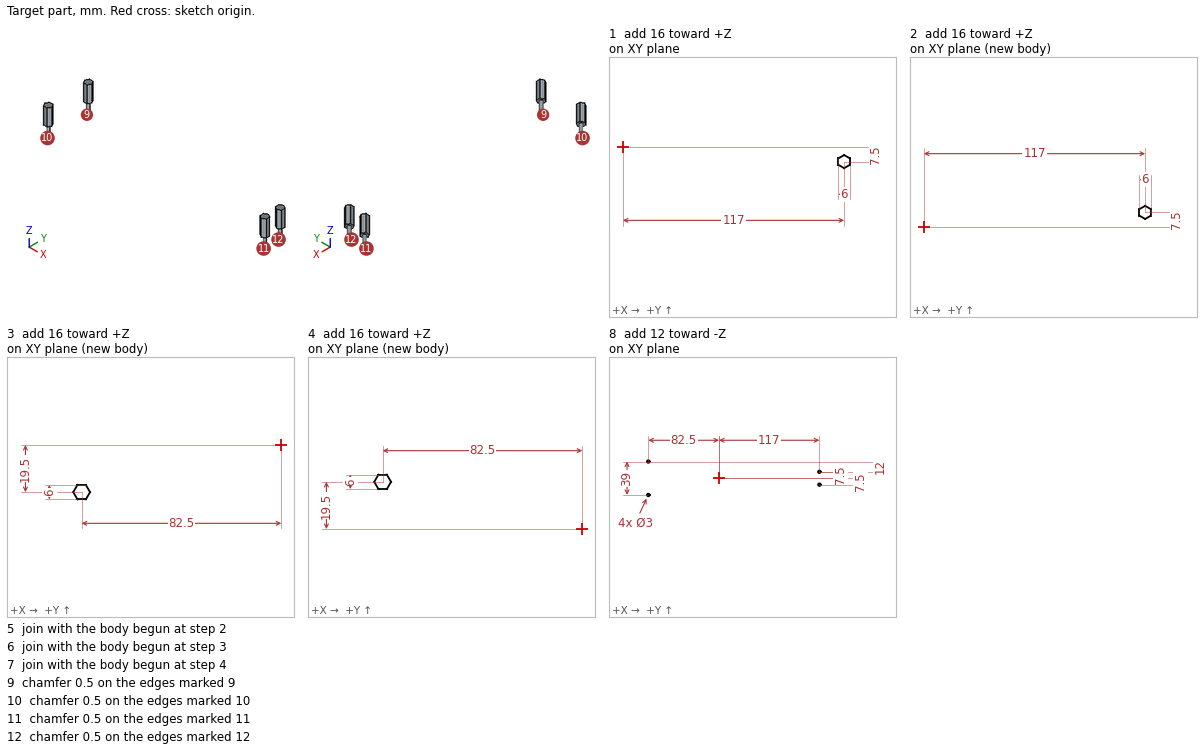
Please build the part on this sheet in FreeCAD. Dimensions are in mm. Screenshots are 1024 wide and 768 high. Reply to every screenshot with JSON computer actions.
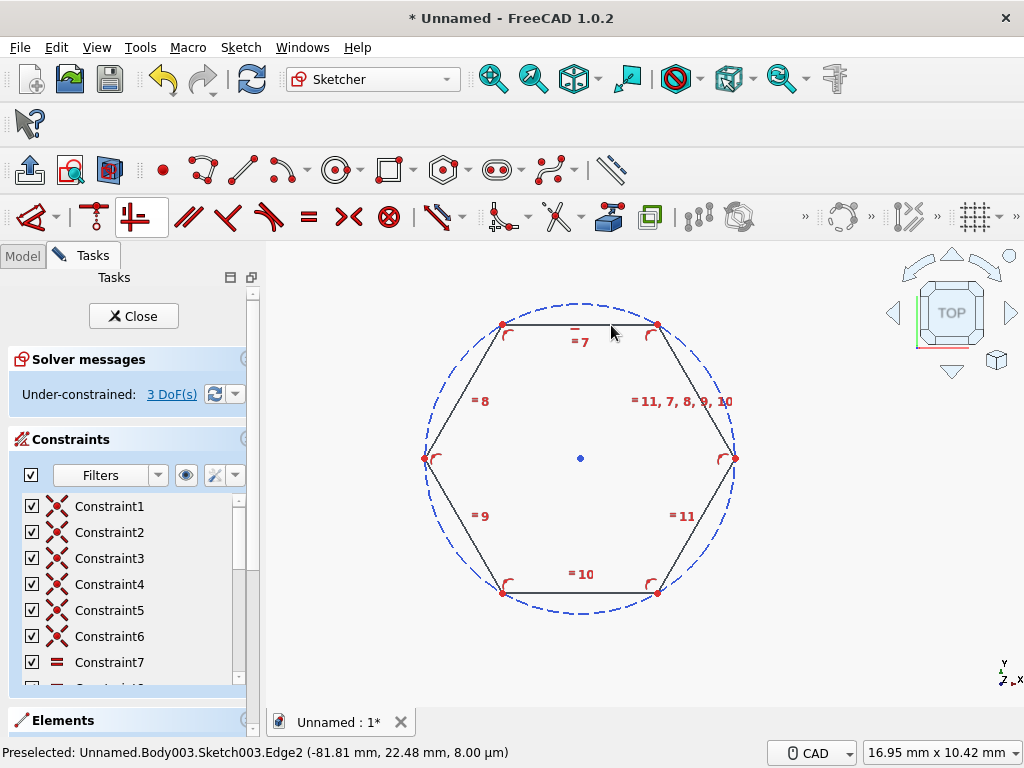
{"action": "left_click", "coordinate": [32, 218]}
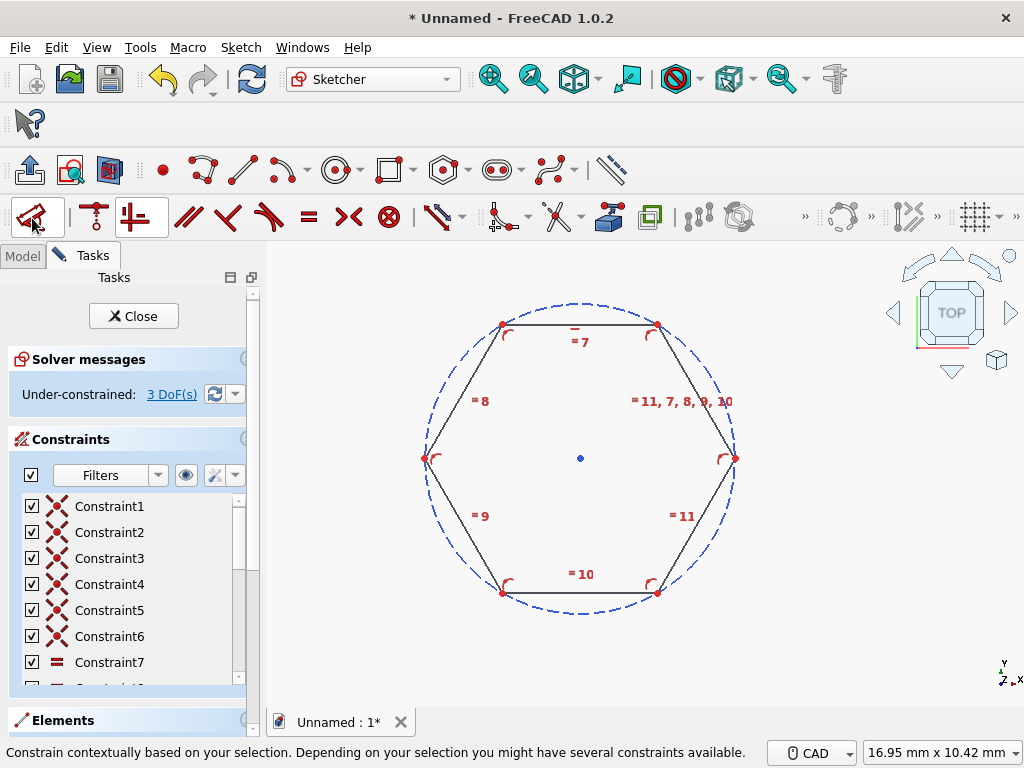
{"action": "left_click", "coordinate": [502, 593]}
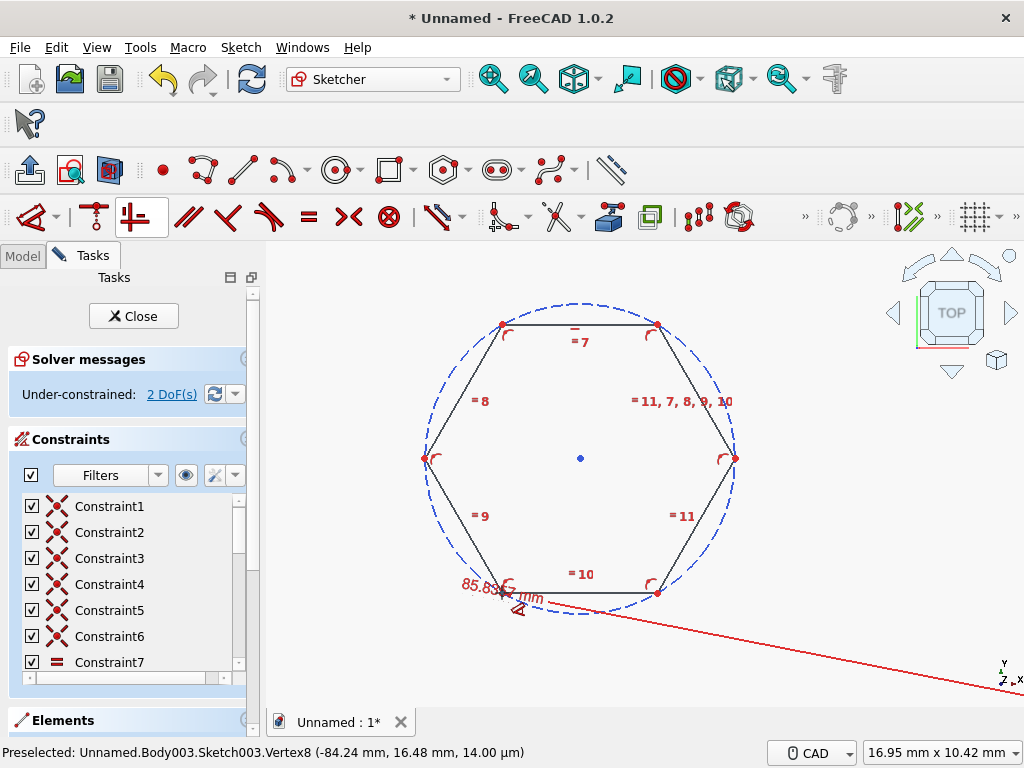
{"action": "left_click", "coordinate": [657, 325]}
{"action": "left_click", "coordinate": [468, 459]}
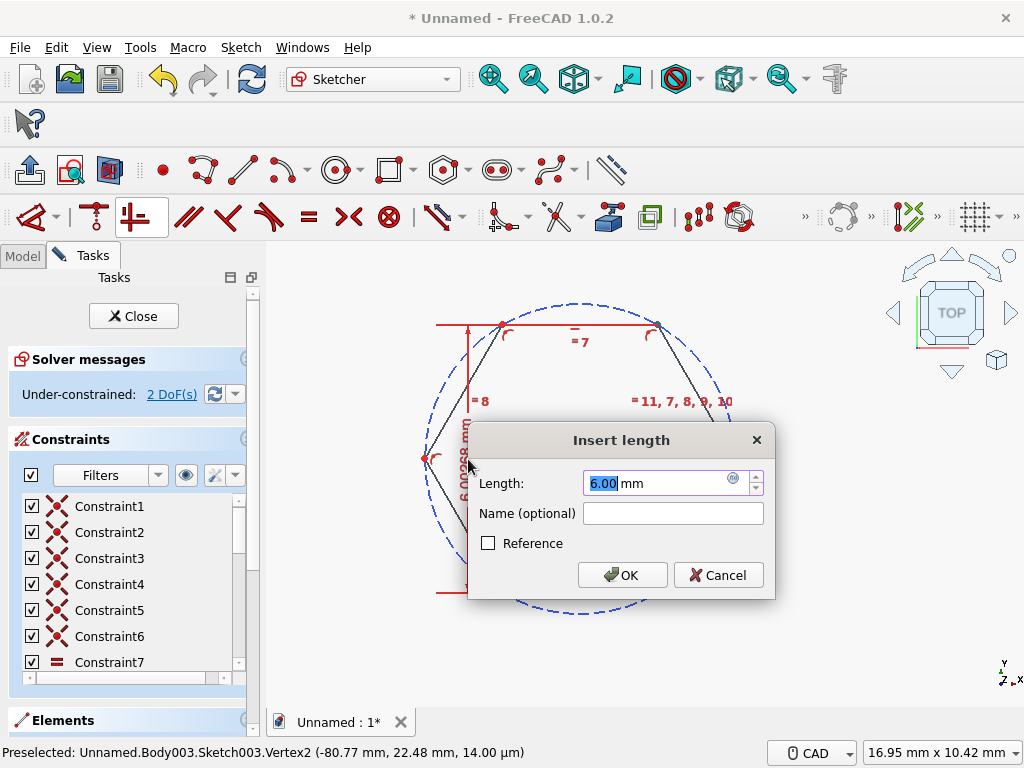
{"action": "type", "text": "6"}
{"action": "key", "text": "Return"}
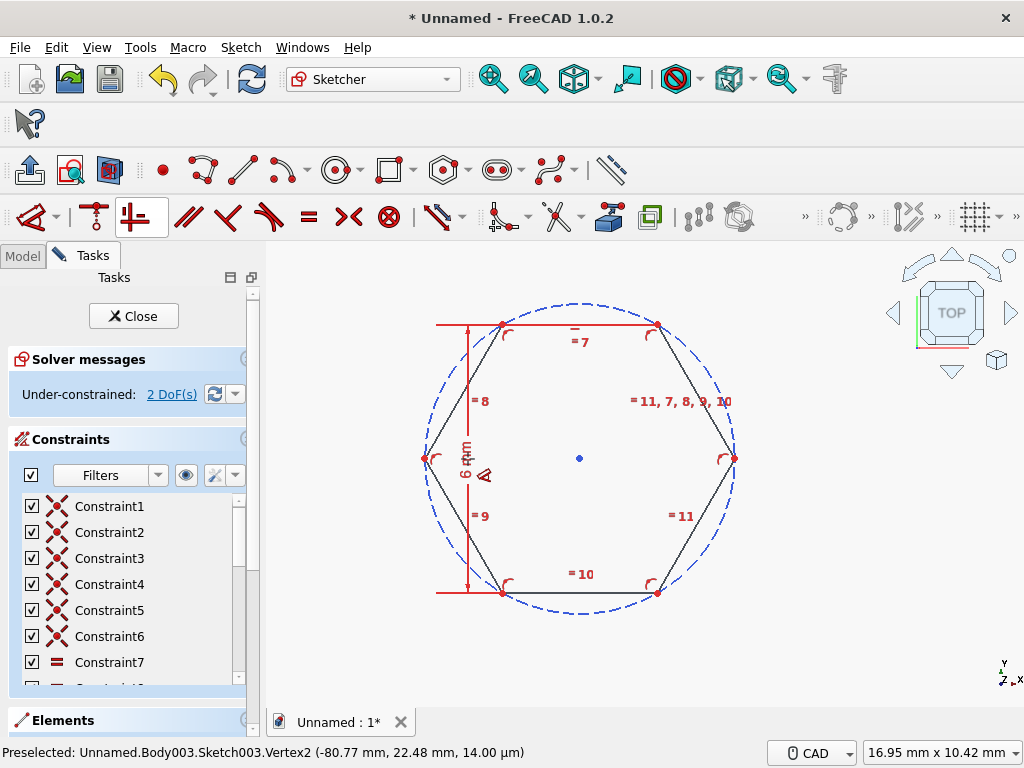
{"action": "left_click", "coordinate": [580, 459]}
{"action": "left_click", "coordinate": [655, 425]}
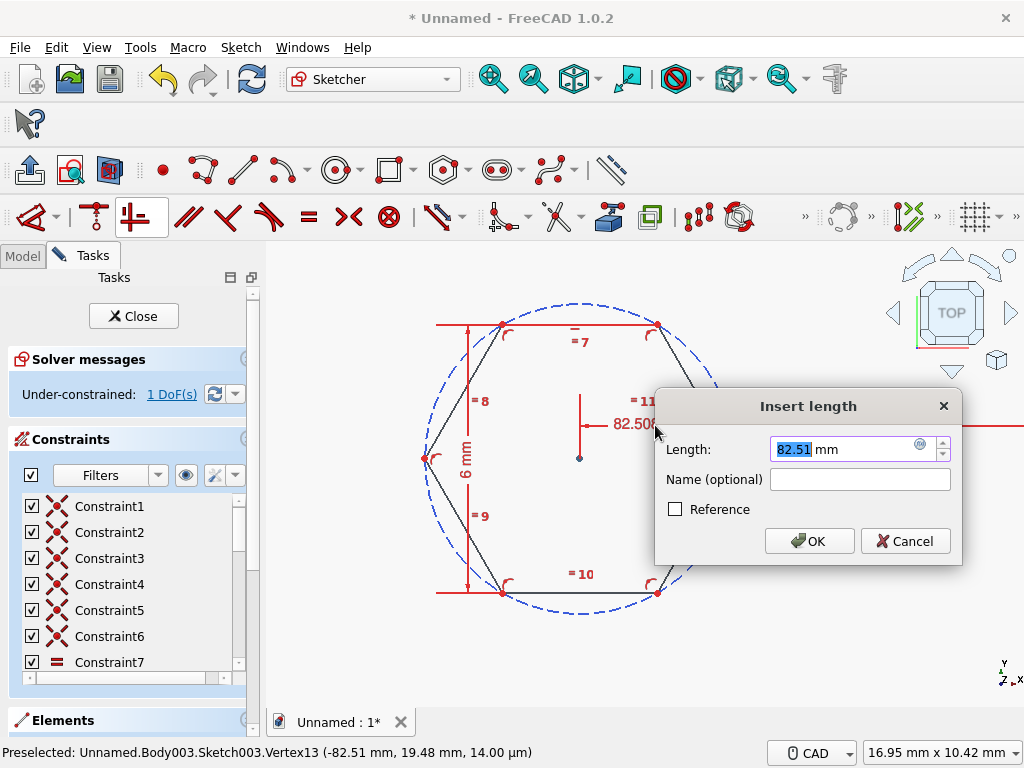
{"action": "type", "text": "82.5"}
{"action": "key", "text": "Return"}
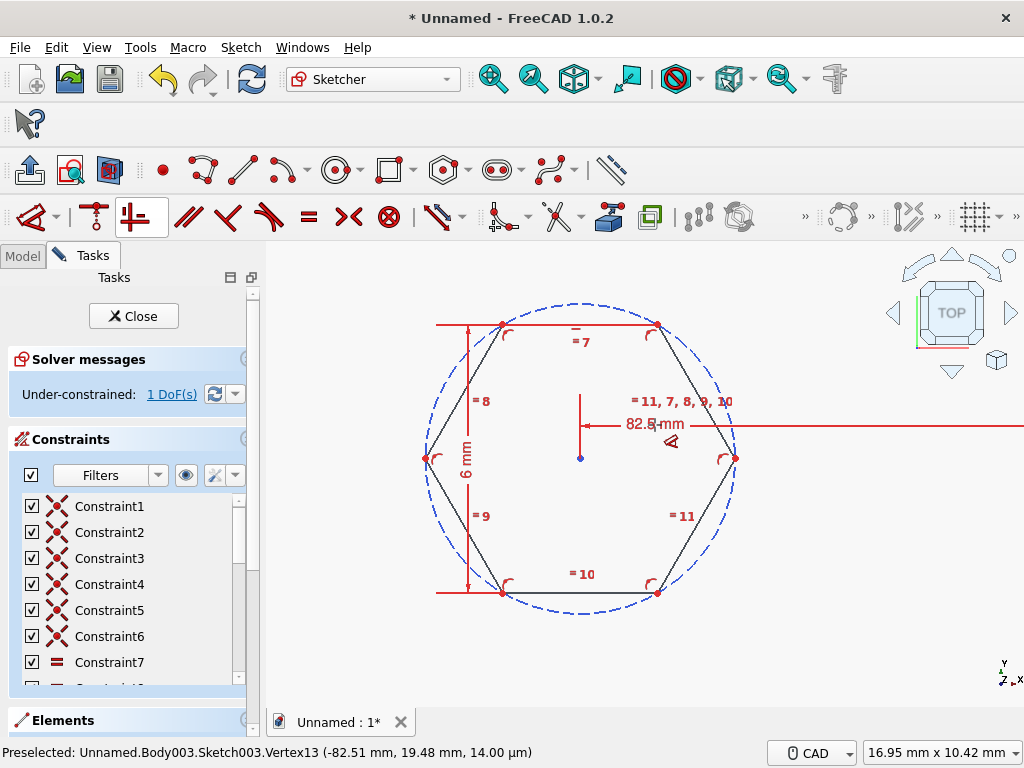
{"action": "left_click", "coordinate": [580, 459]}
{"action": "left_click", "coordinate": [546, 569]}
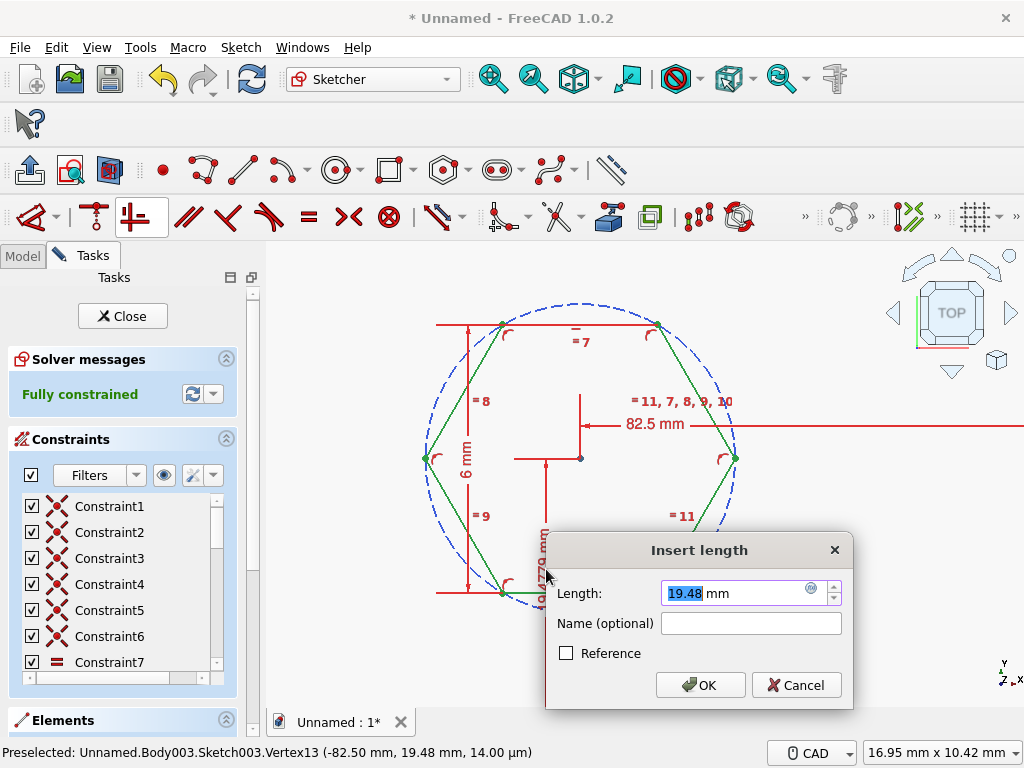
{"action": "type", "text": "19.5"}
{"action": "key", "text": "Return"}
{"action": "key", "text": "Escape"}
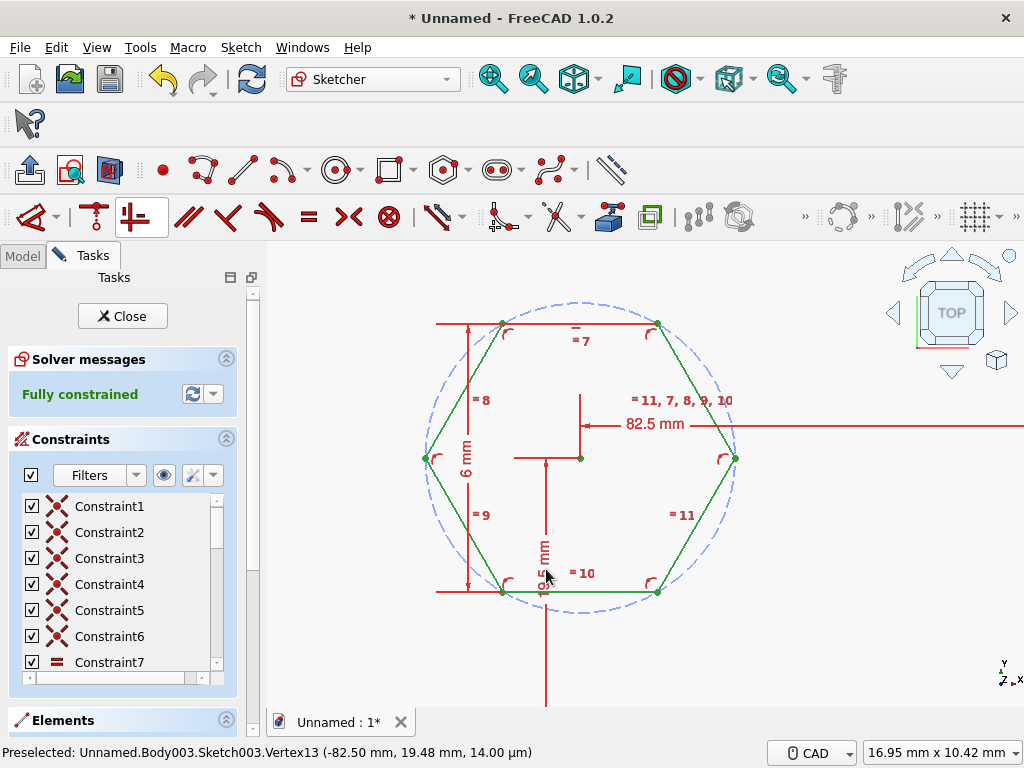
{"action": "left_click", "coordinate": [123, 316]}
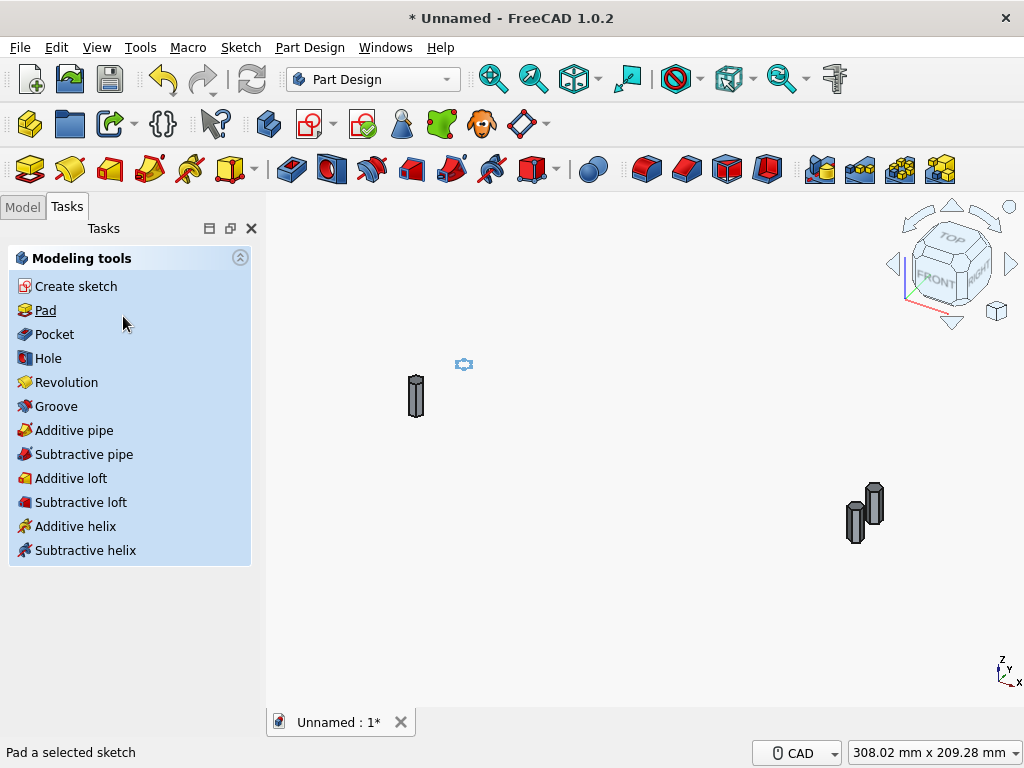
{"action": "left_click", "coordinate": [30, 170]}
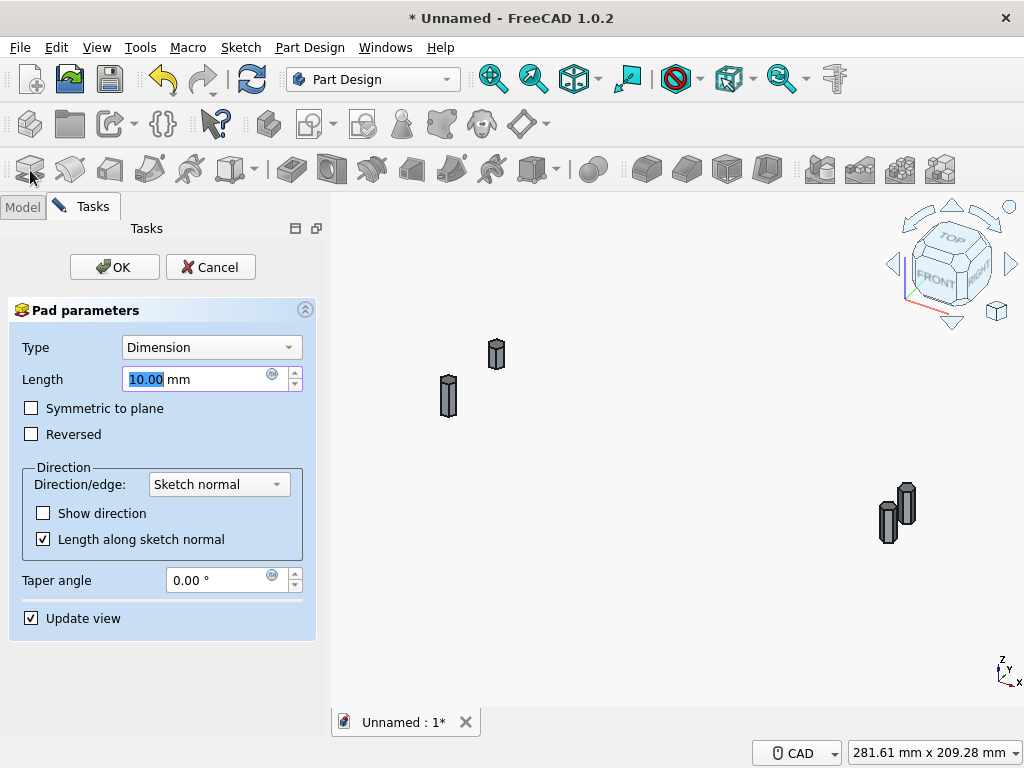
{"action": "type", "text": "16"}
{"action": "key", "text": "Tab"}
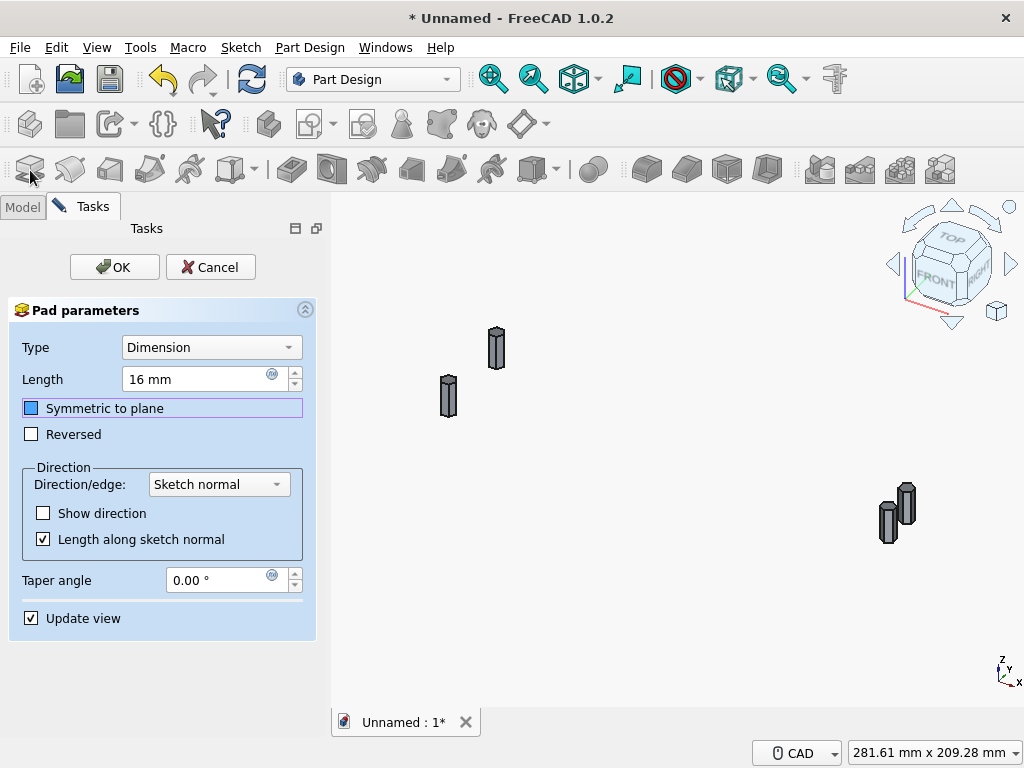
{"action": "left_click", "coordinate": [115, 267]}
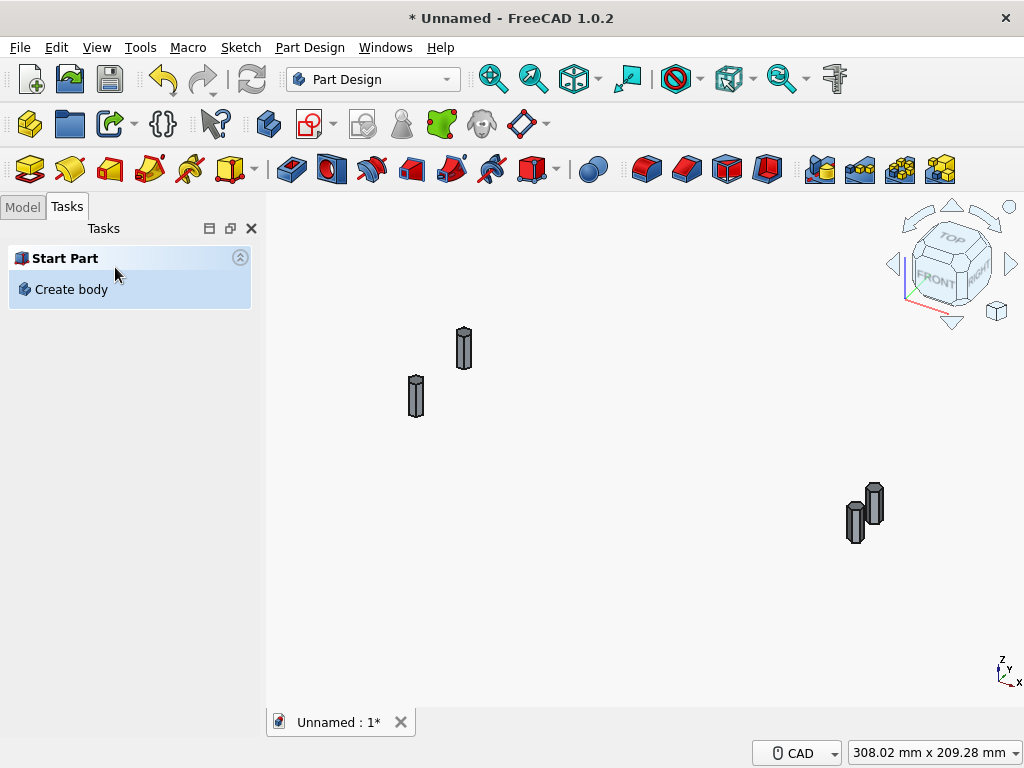
{"action": "left_click", "coordinate": [494, 80]}